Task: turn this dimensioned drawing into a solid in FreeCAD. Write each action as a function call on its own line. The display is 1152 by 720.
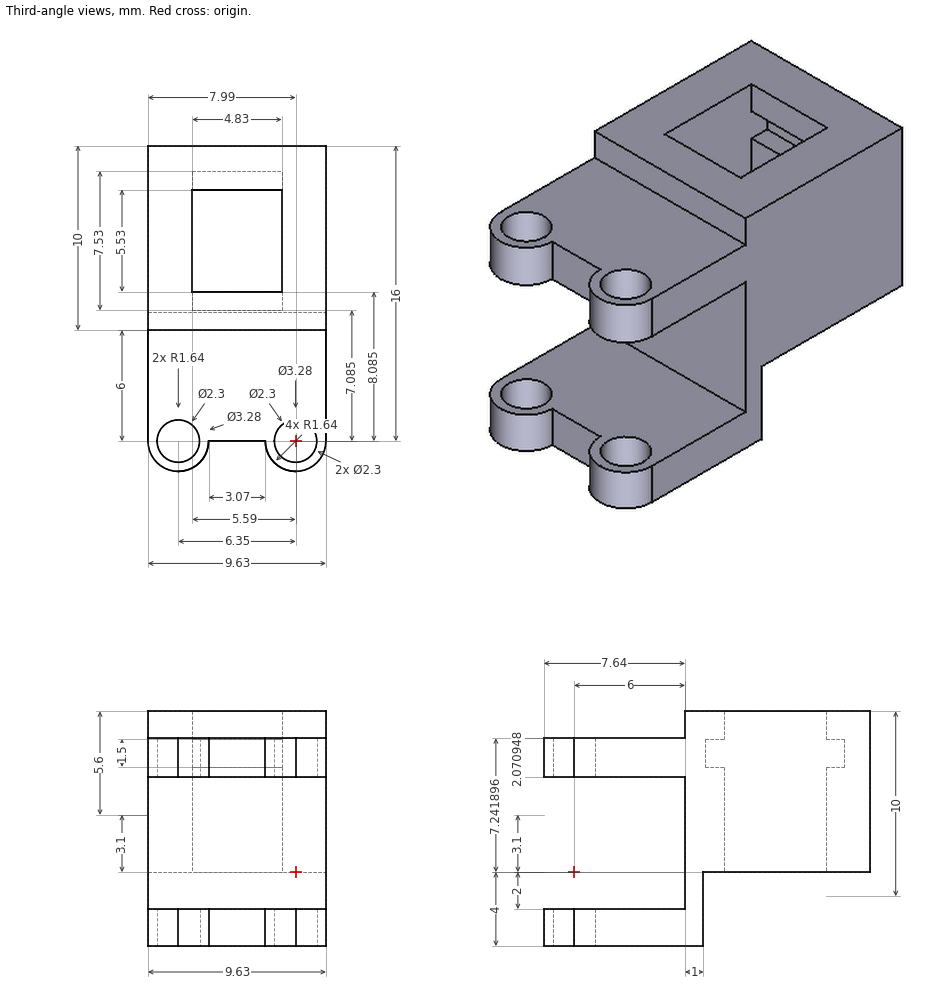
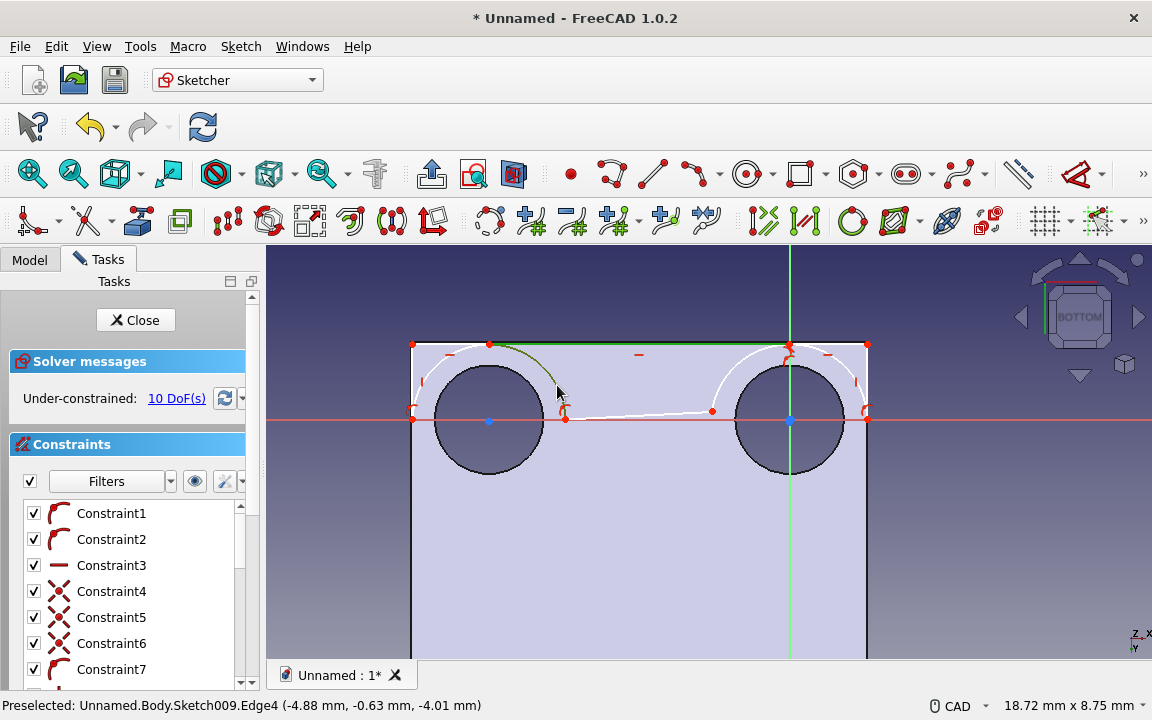
key(t)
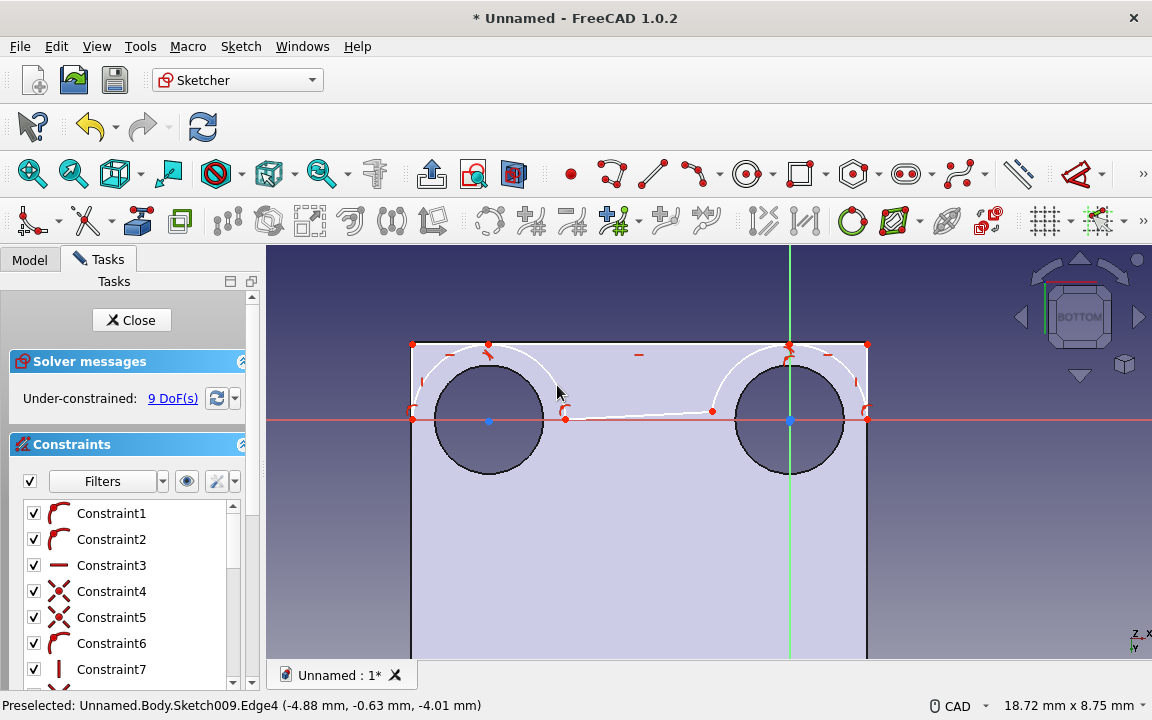
click(699, 344)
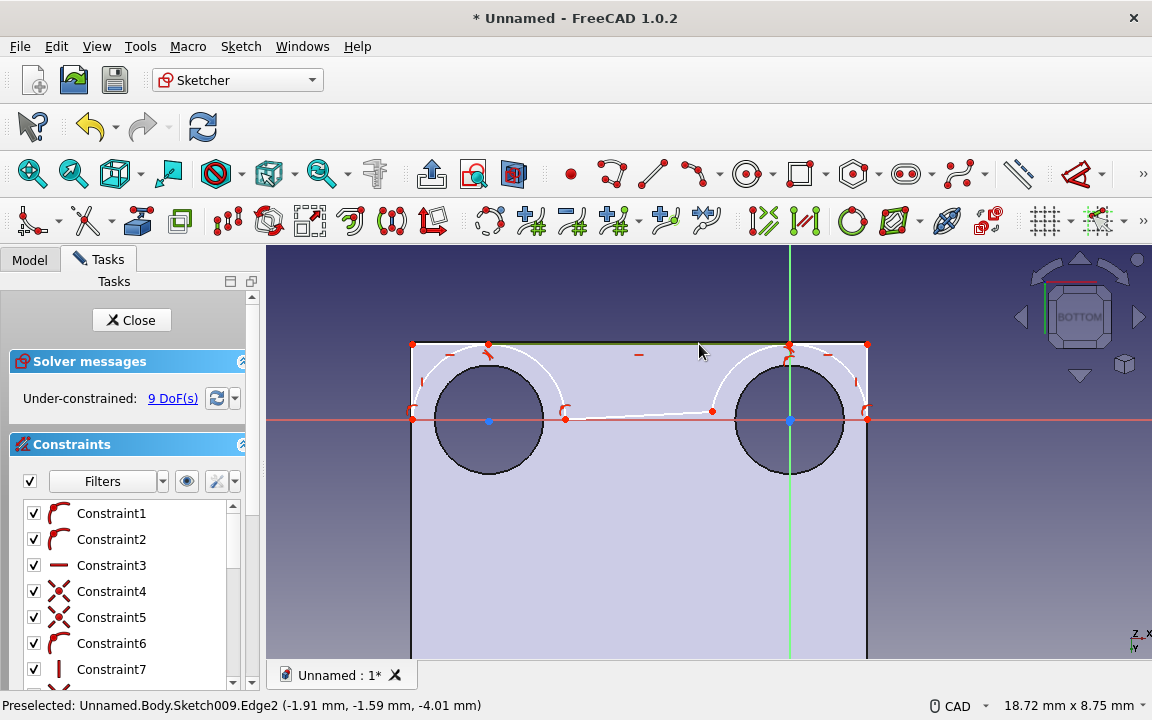
click(844, 366)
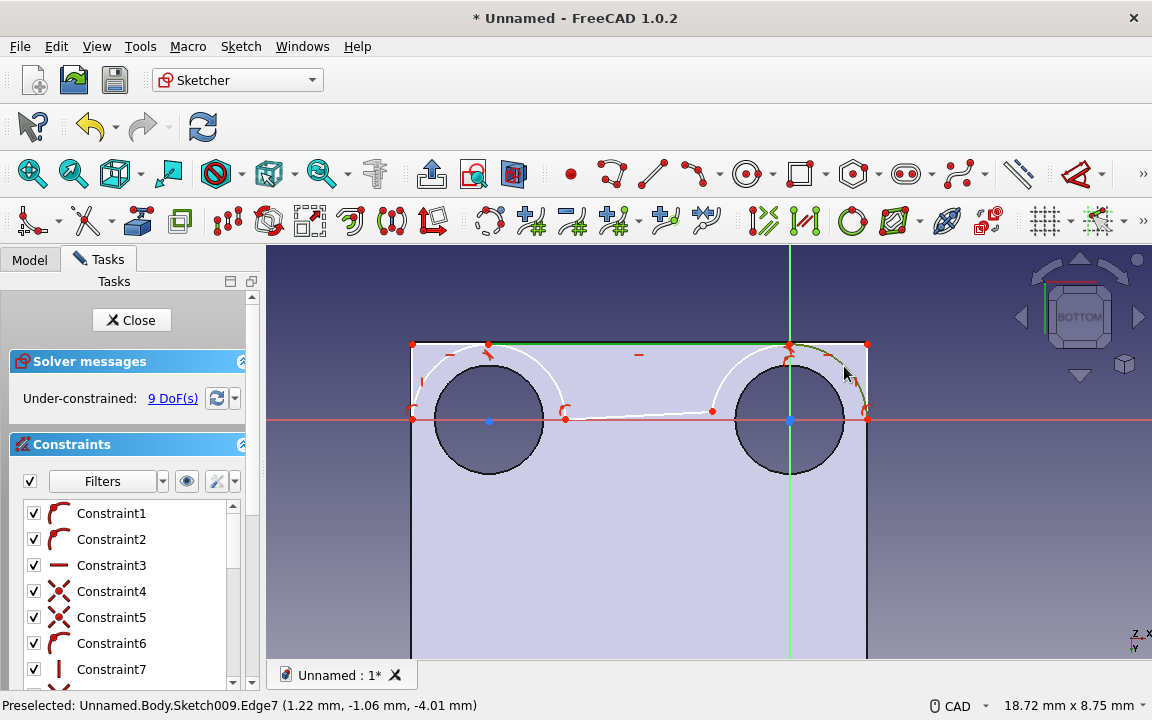
key(t)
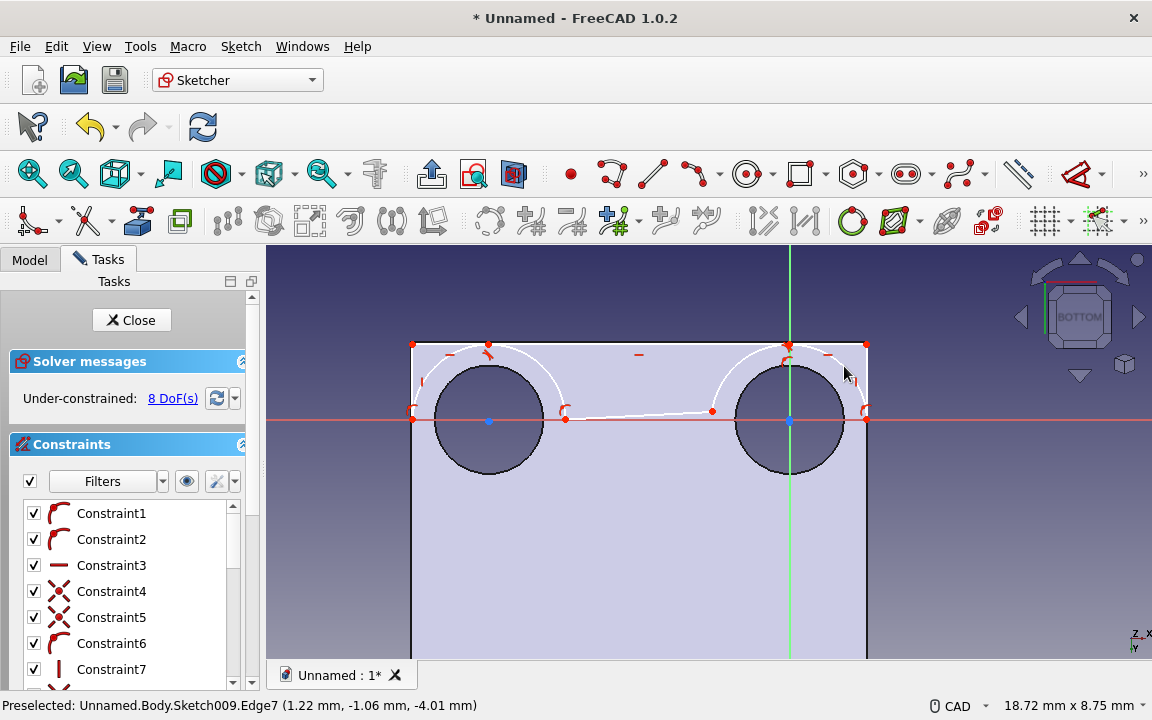
click(699, 344)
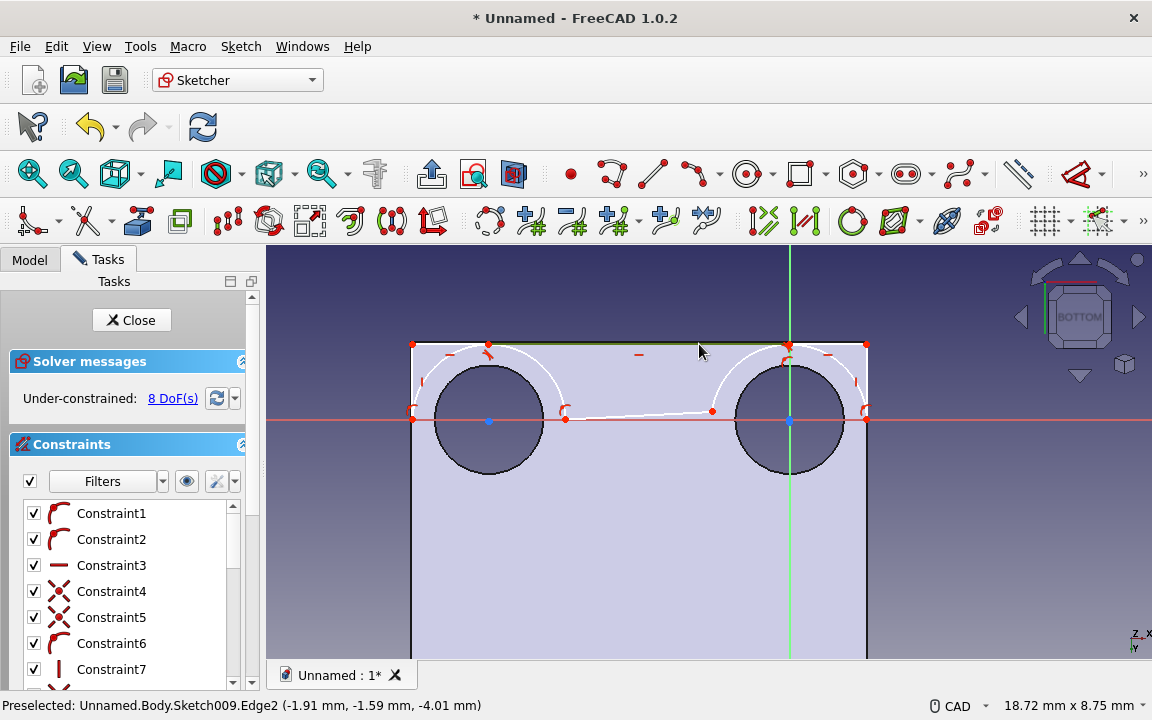
click(435, 367)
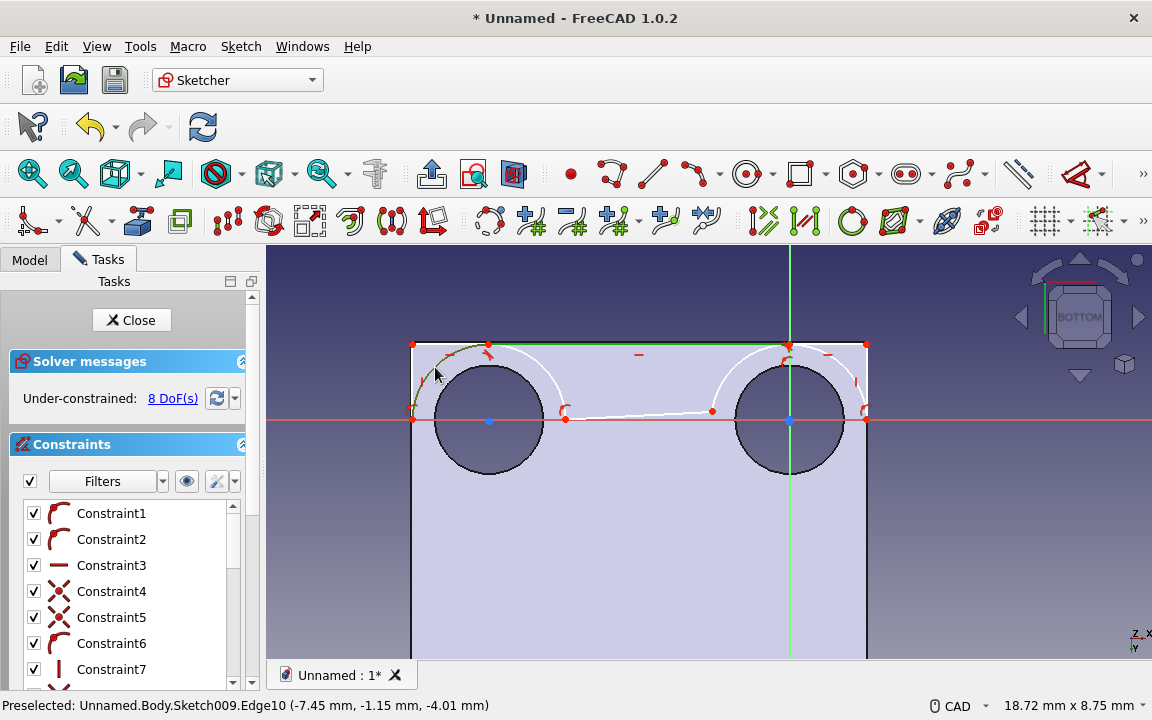
key(t)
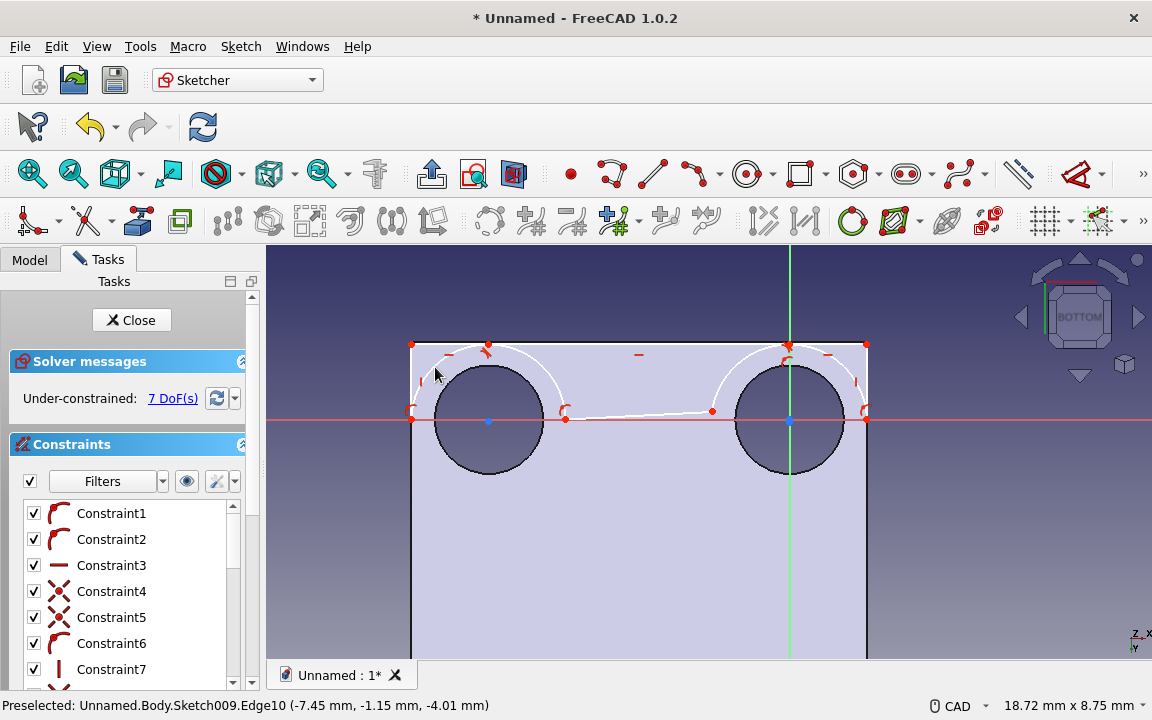
click(867, 367)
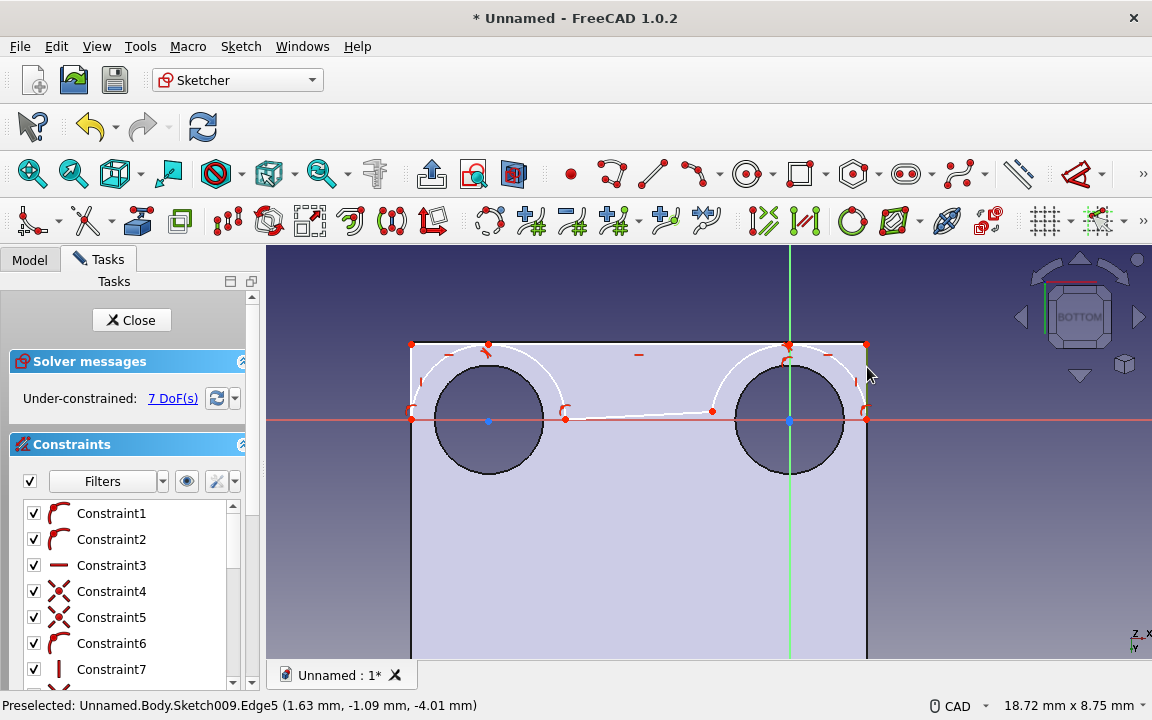
scroll(858, 385, up, 3)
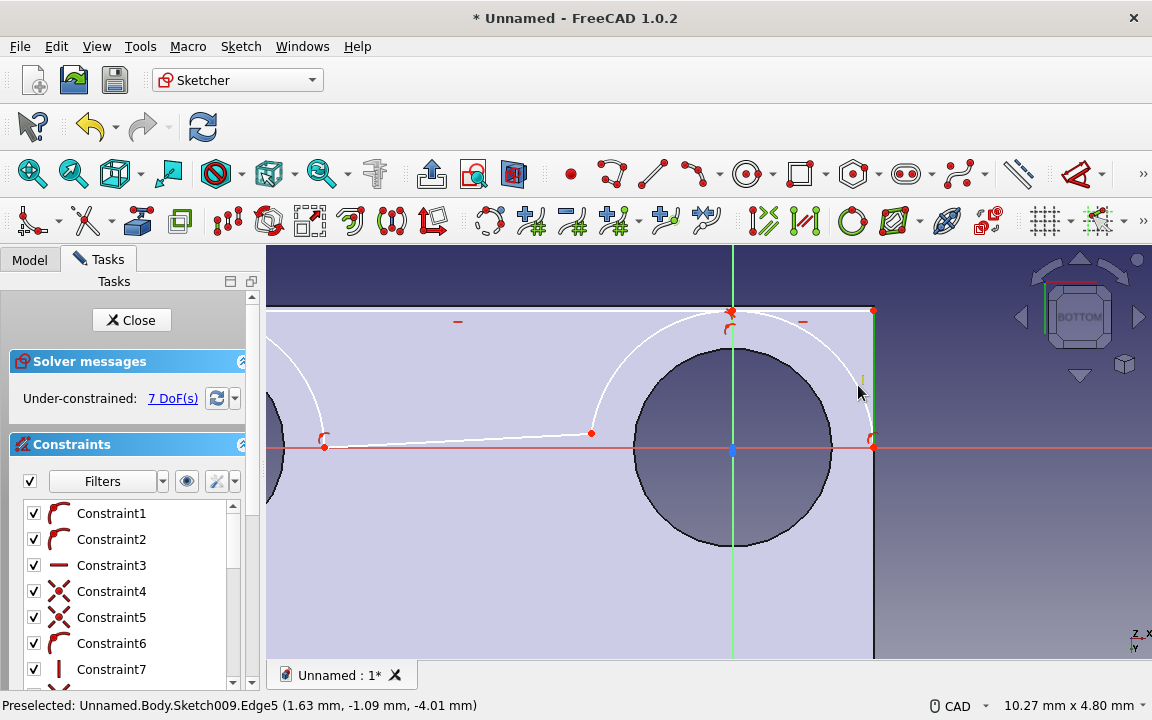
click(857, 385)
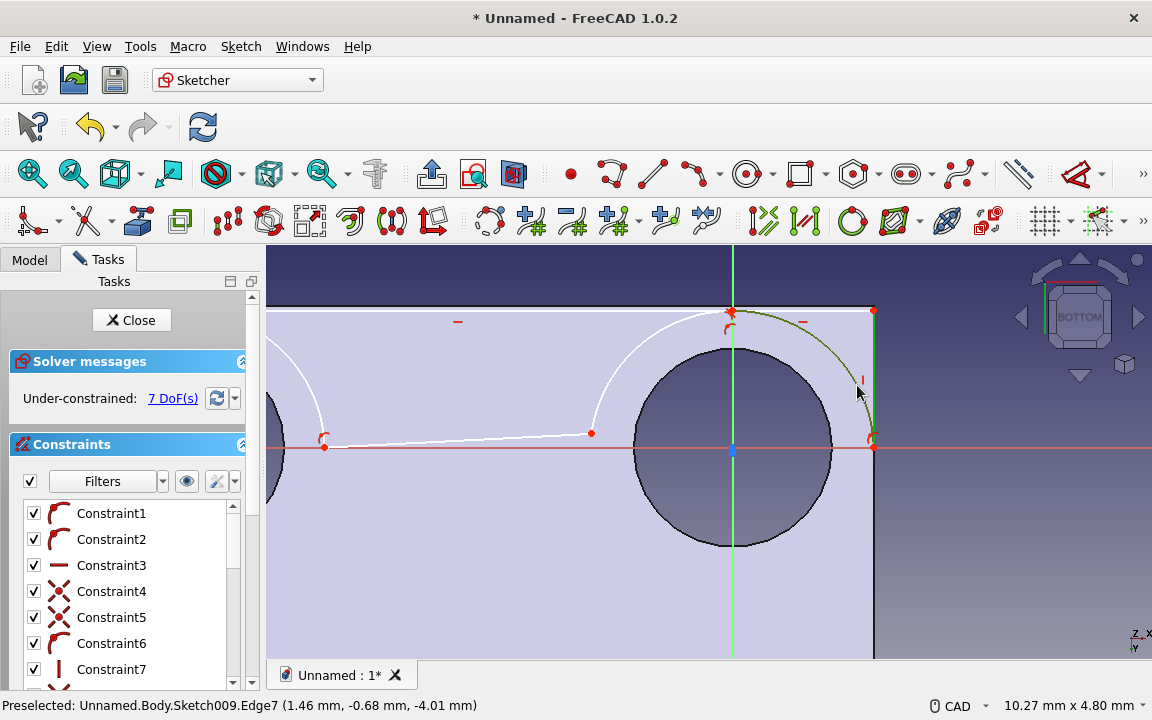
key(t)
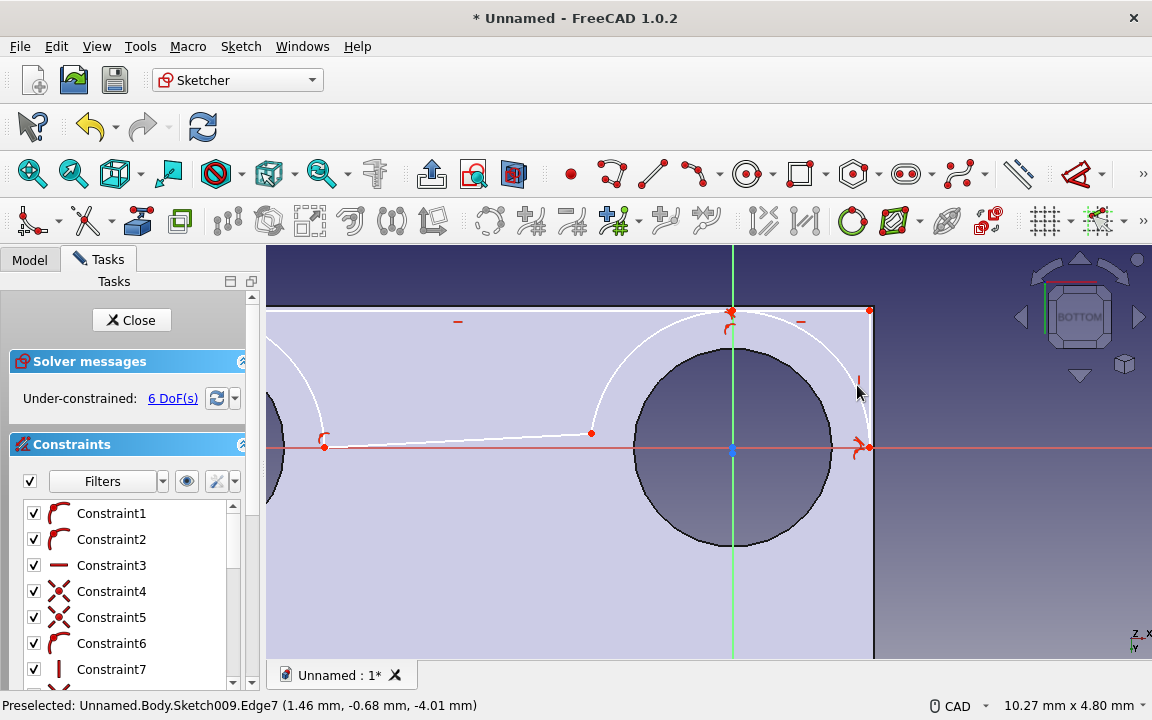
scroll(861, 543, down, 3)